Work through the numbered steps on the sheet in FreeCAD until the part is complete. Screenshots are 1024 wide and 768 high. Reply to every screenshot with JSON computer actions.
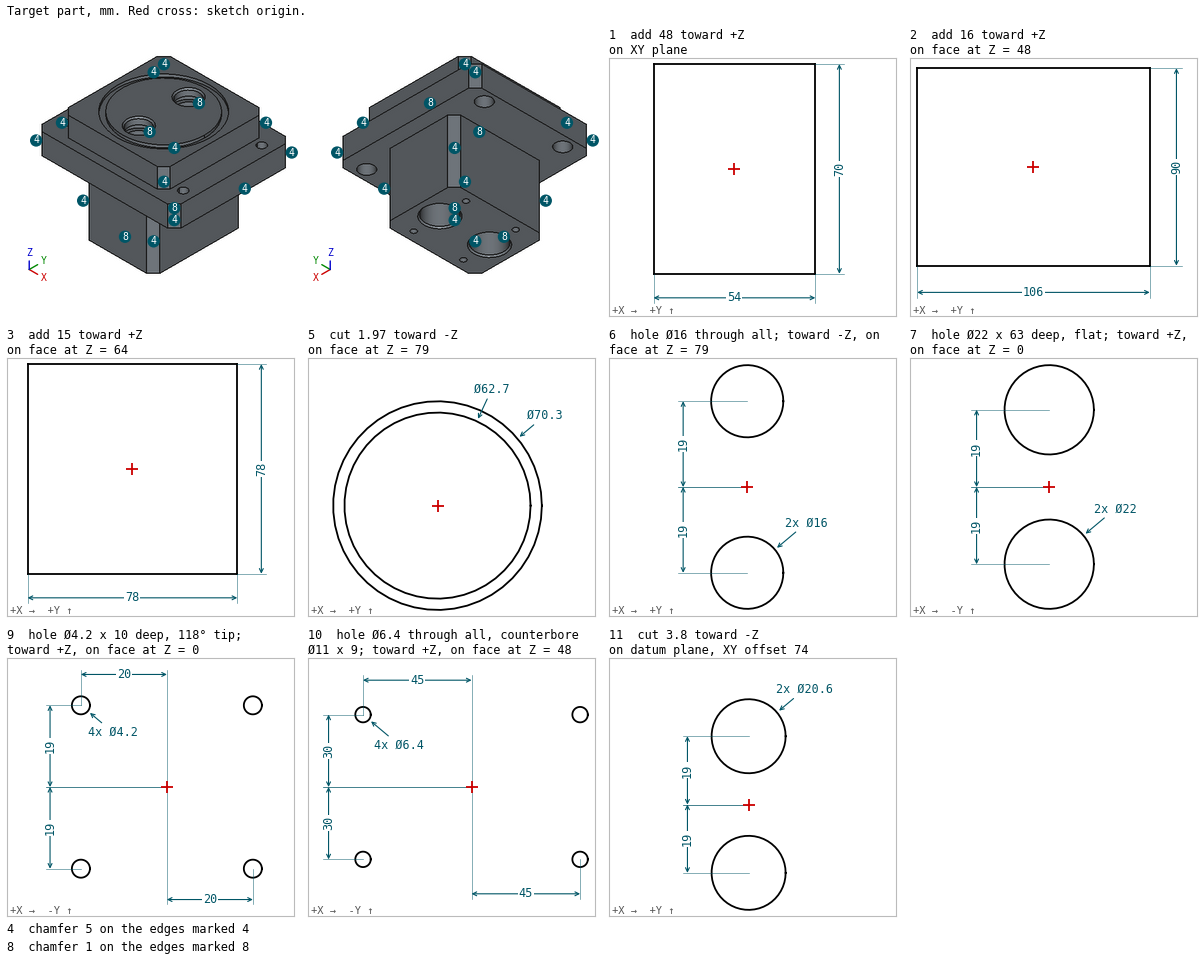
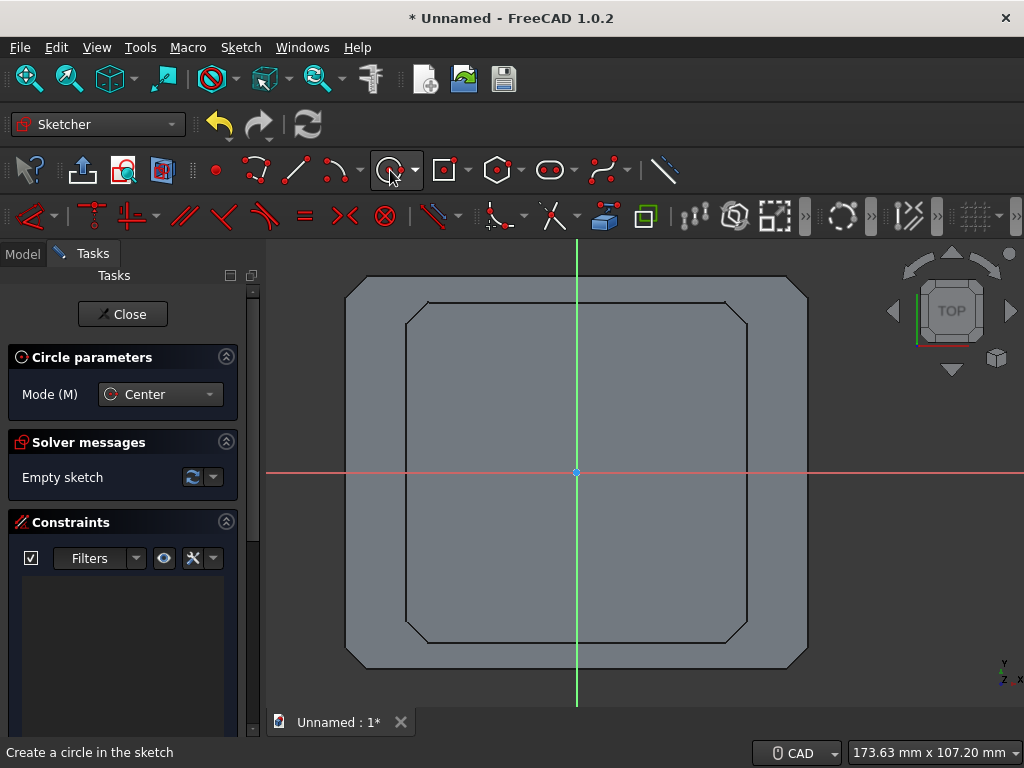
{"action": "left_click", "coordinate": [577, 473]}
{"action": "mouse_move", "coordinate": [685, 364]}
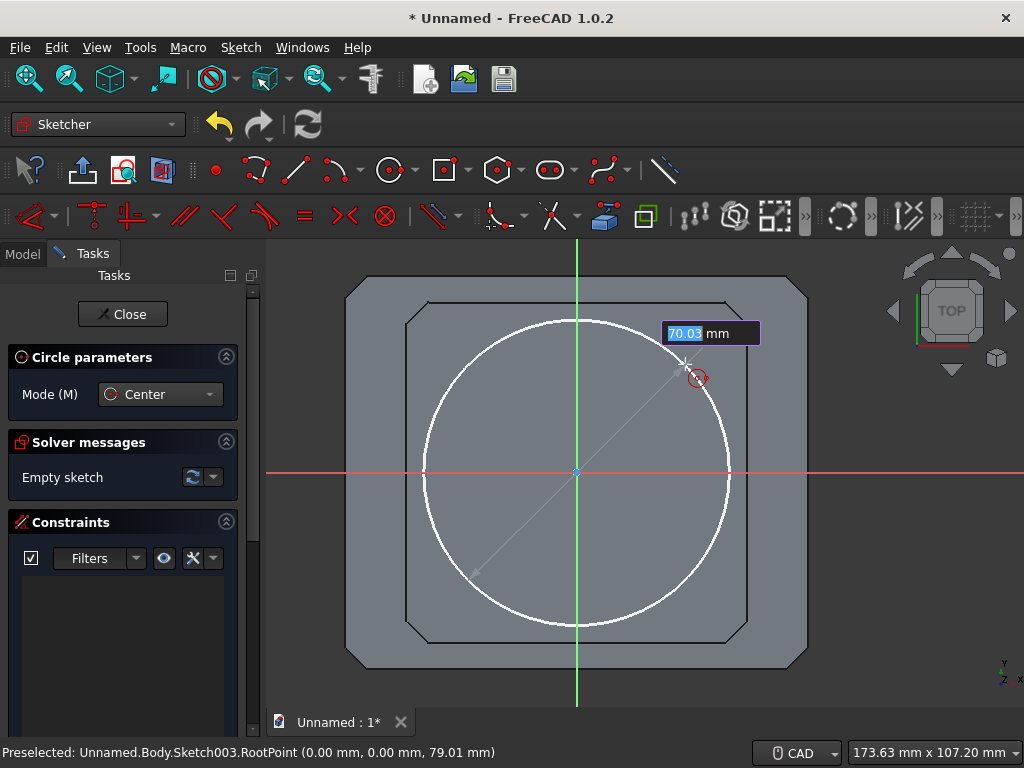
{"action": "type", "text": "70.3"}
{"action": "key", "text": "Return"}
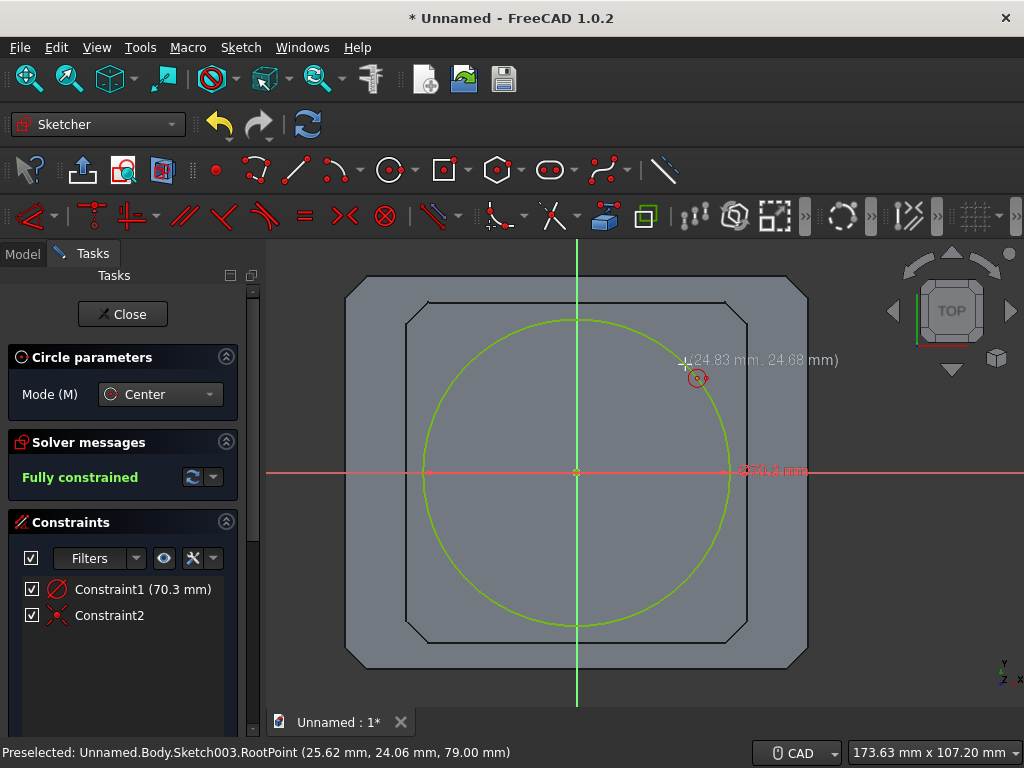
{"action": "left_click", "coordinate": [577, 473]}
{"action": "mouse_move", "coordinate": [673, 376]}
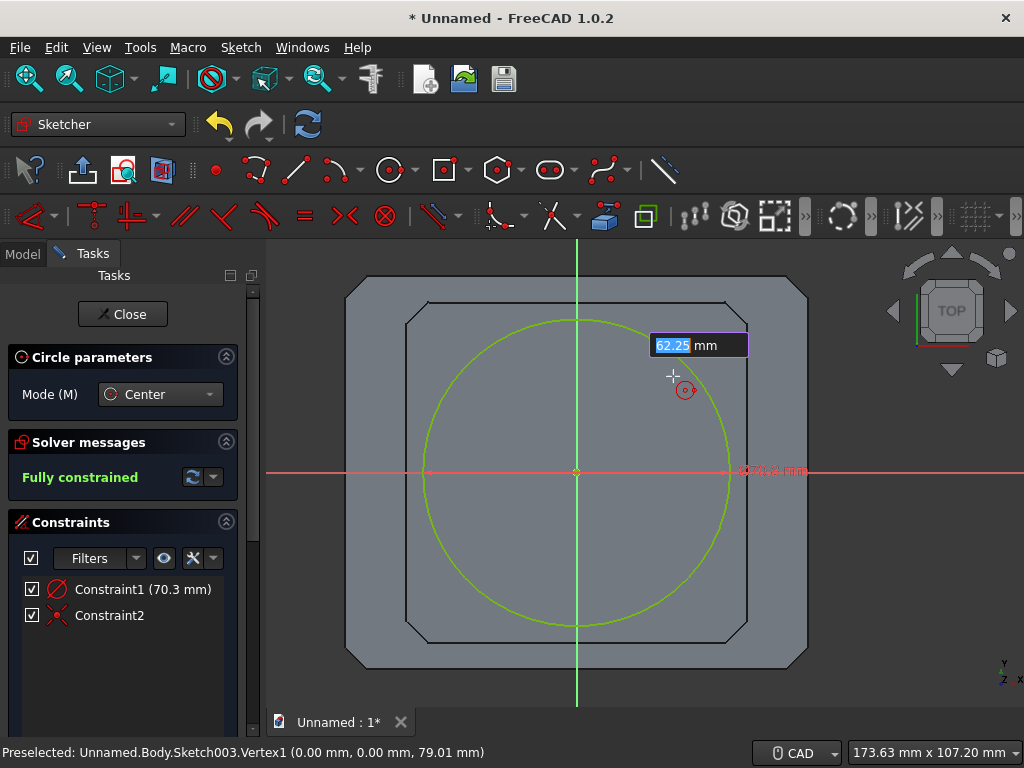
{"action": "type", "text": "62.7"}
{"action": "key", "text": "Return"}
{"action": "key", "text": "Escape"}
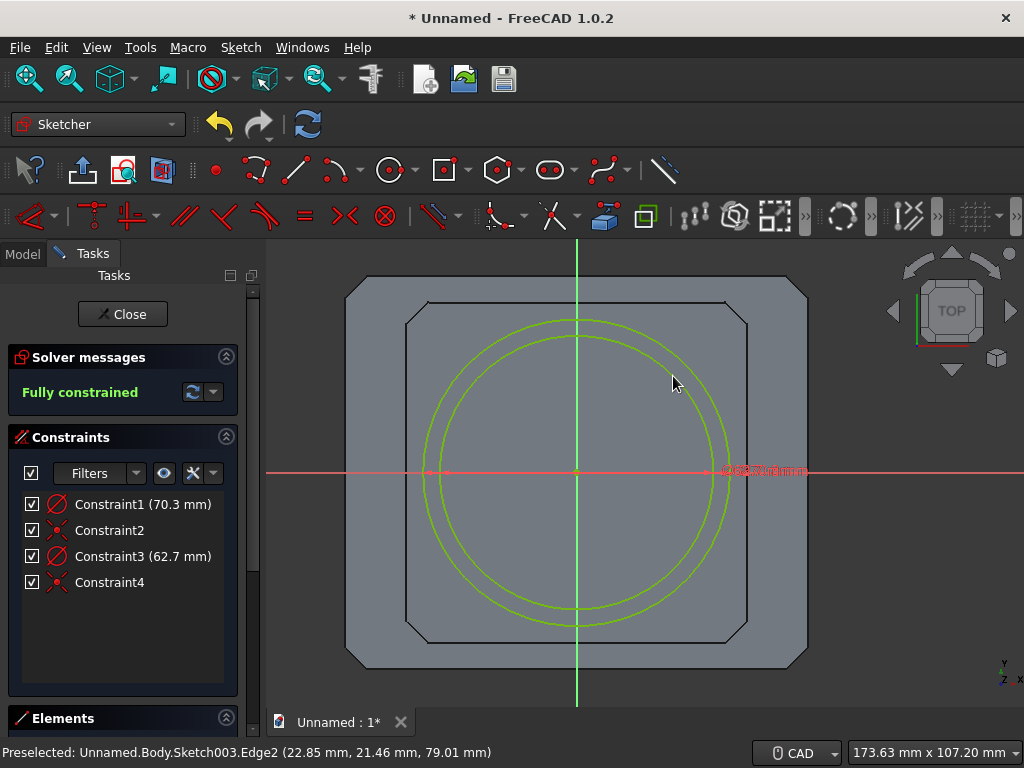
{"action": "left_click", "coordinate": [123, 314]}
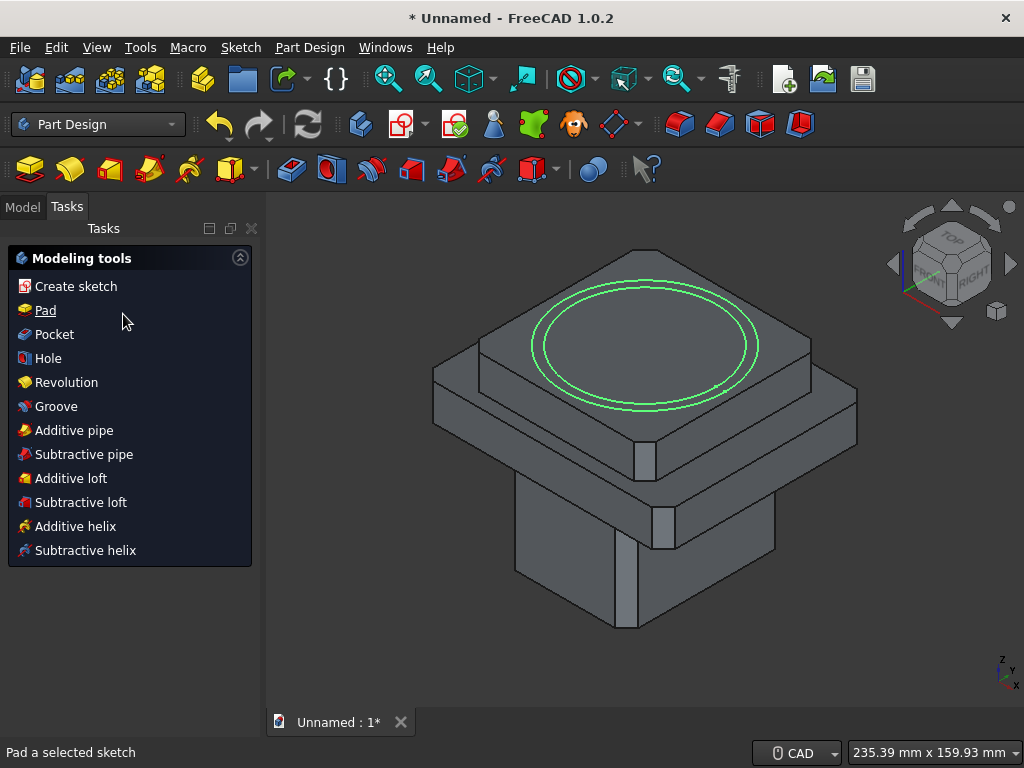
{"action": "left_click", "coordinate": [292, 170]}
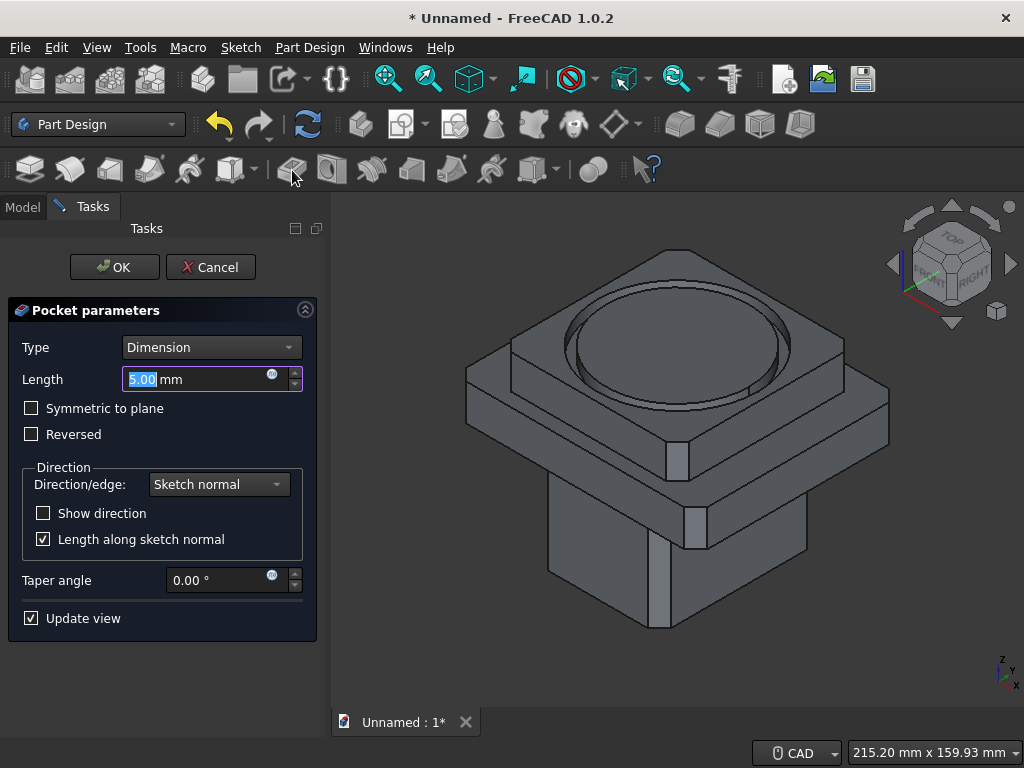
{"action": "type", "text": "1.97"}
{"action": "key", "text": "Tab"}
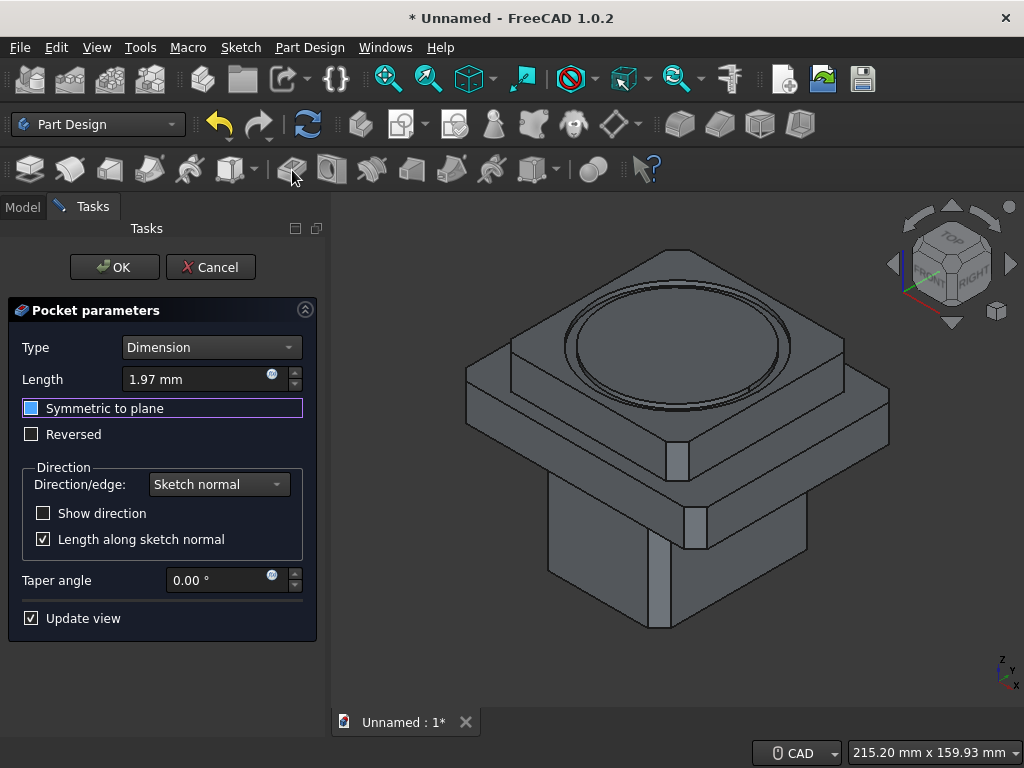
{"action": "left_click", "coordinate": [115, 267]}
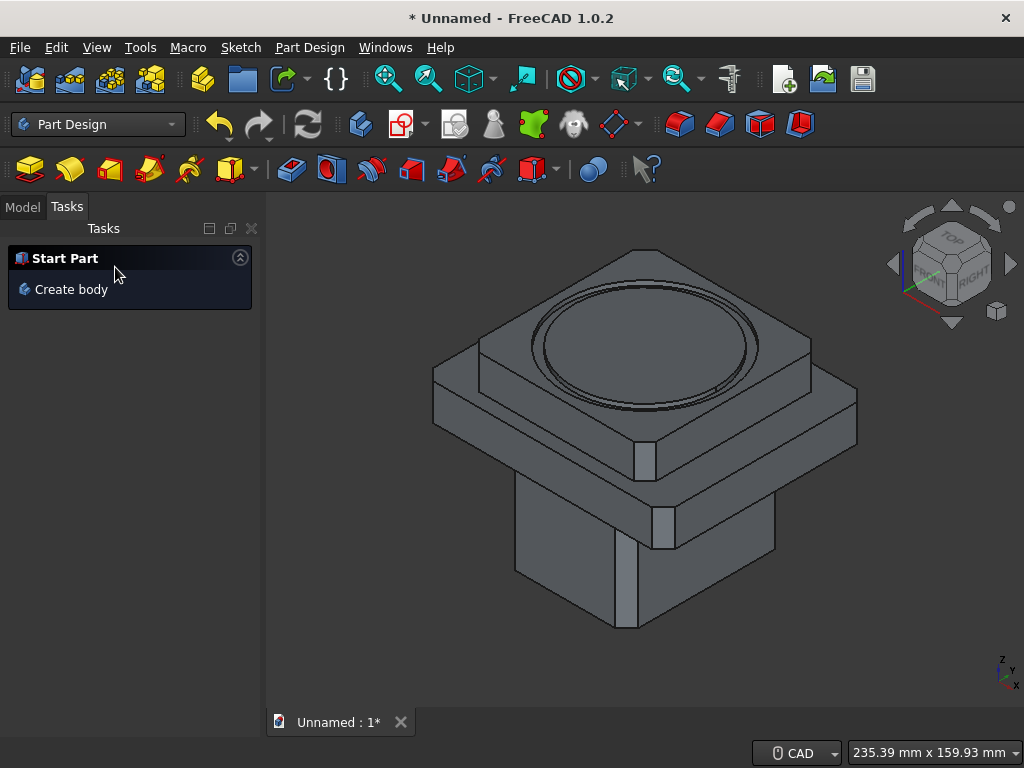
{"action": "left_click", "coordinate": [645, 345]}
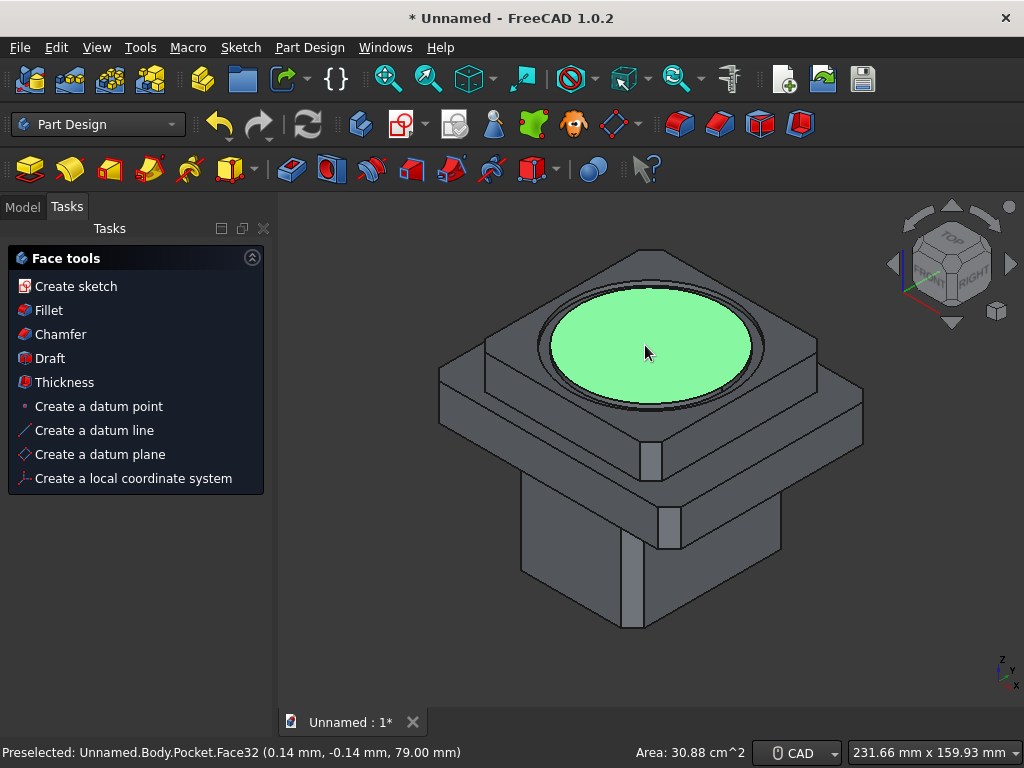
{"action": "left_click", "coordinate": [402, 124]}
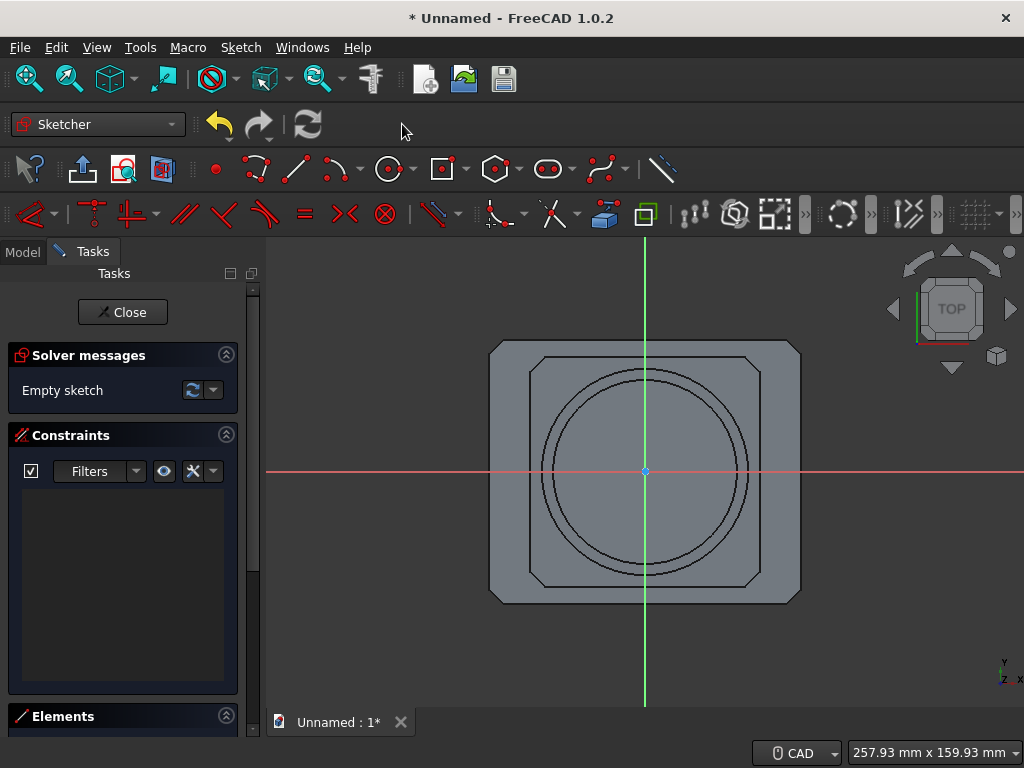
{"action": "scroll", "coordinate": [728, 472], "scroll_direction": "up", "scroll_amount": 3}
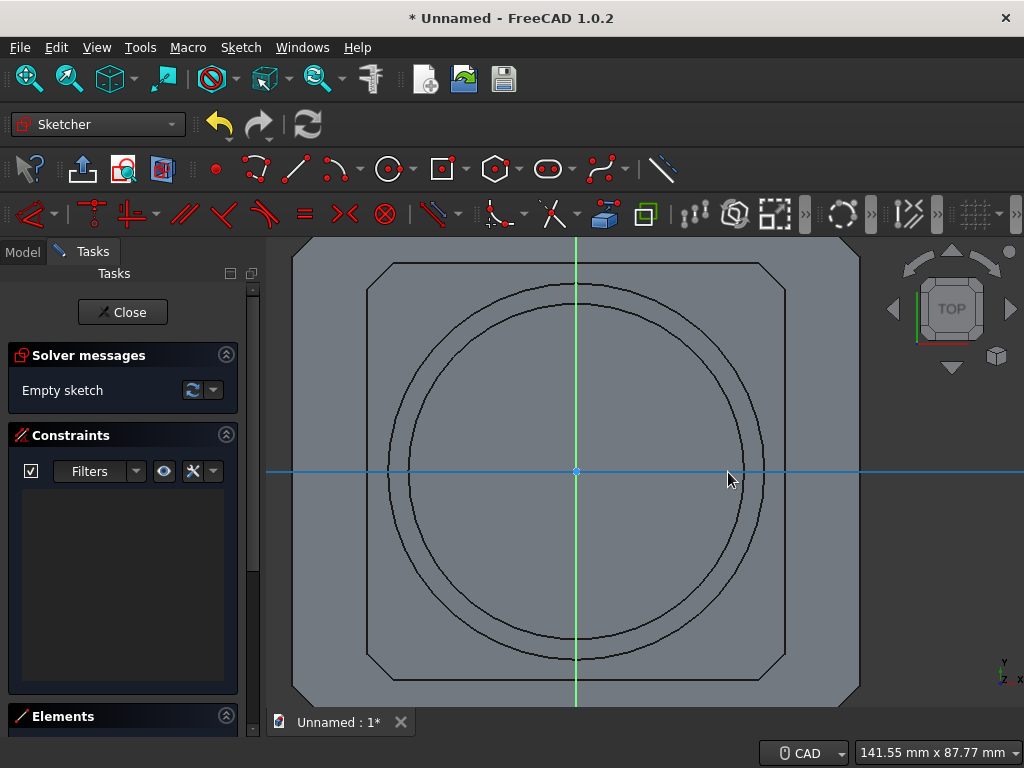
{"action": "left_click", "coordinate": [390, 170]}